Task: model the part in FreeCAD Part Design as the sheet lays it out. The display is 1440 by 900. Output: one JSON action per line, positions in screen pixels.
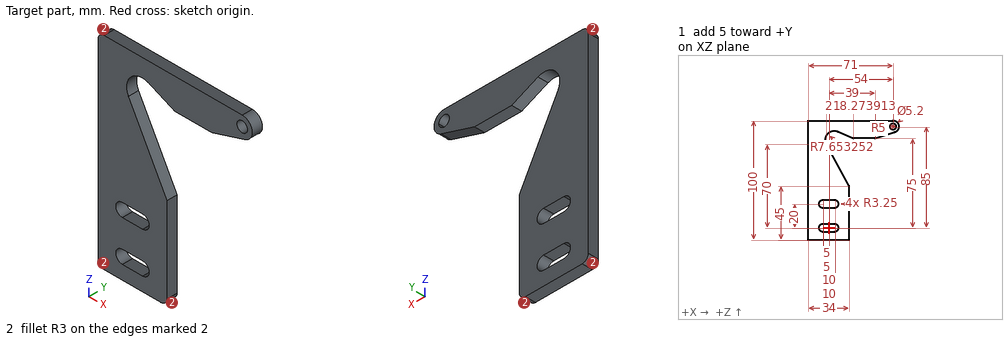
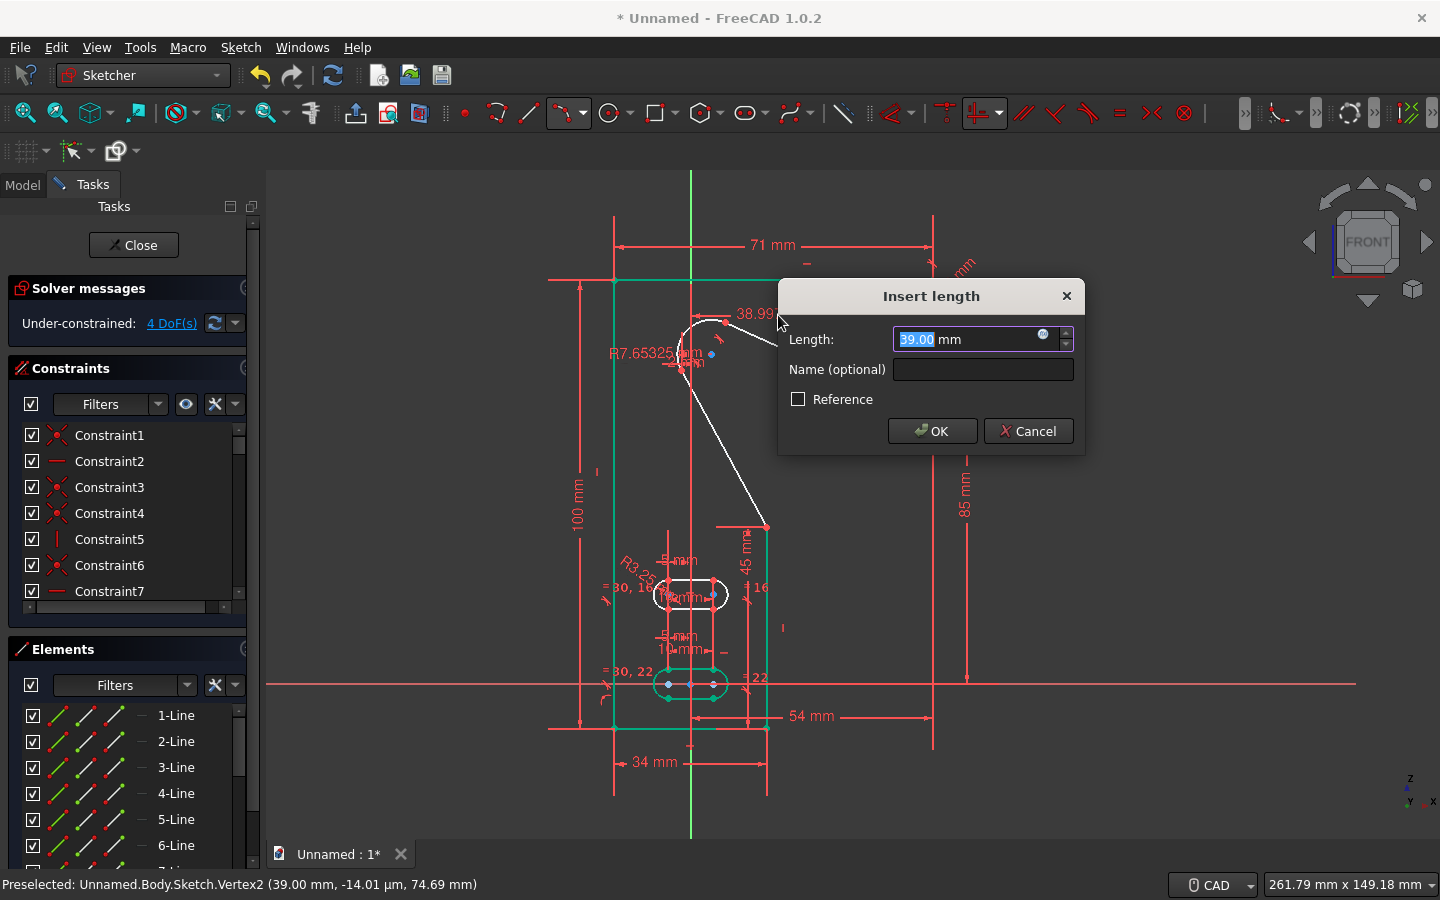
{"action": "type", "text": "39"}
{"action": "key", "text": "Return"}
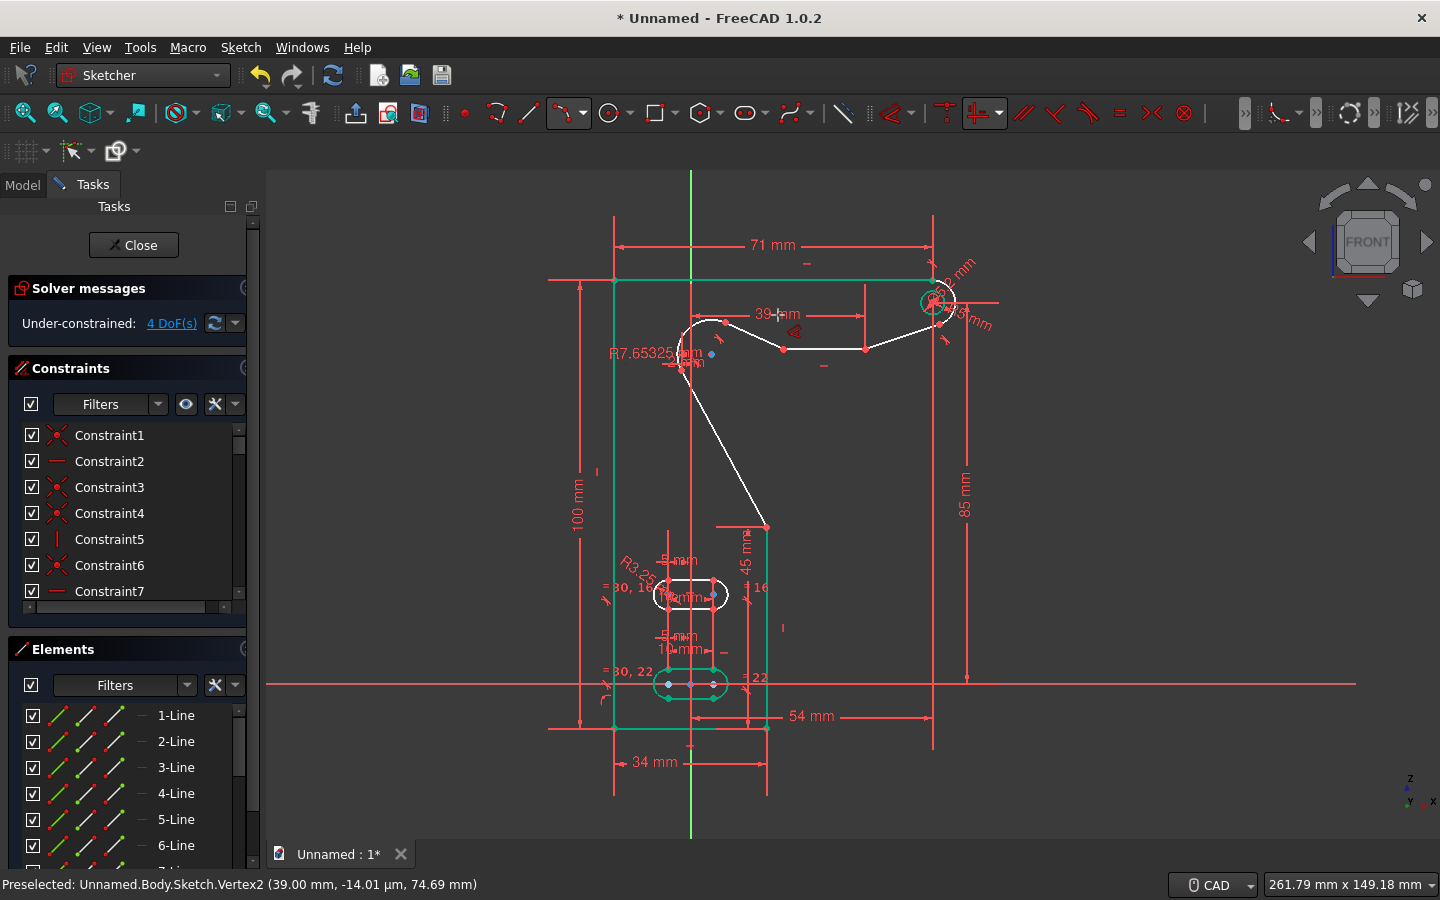
{"action": "left_click", "coordinate": [865, 349]}
{"action": "left_click", "coordinate": [657, 517]}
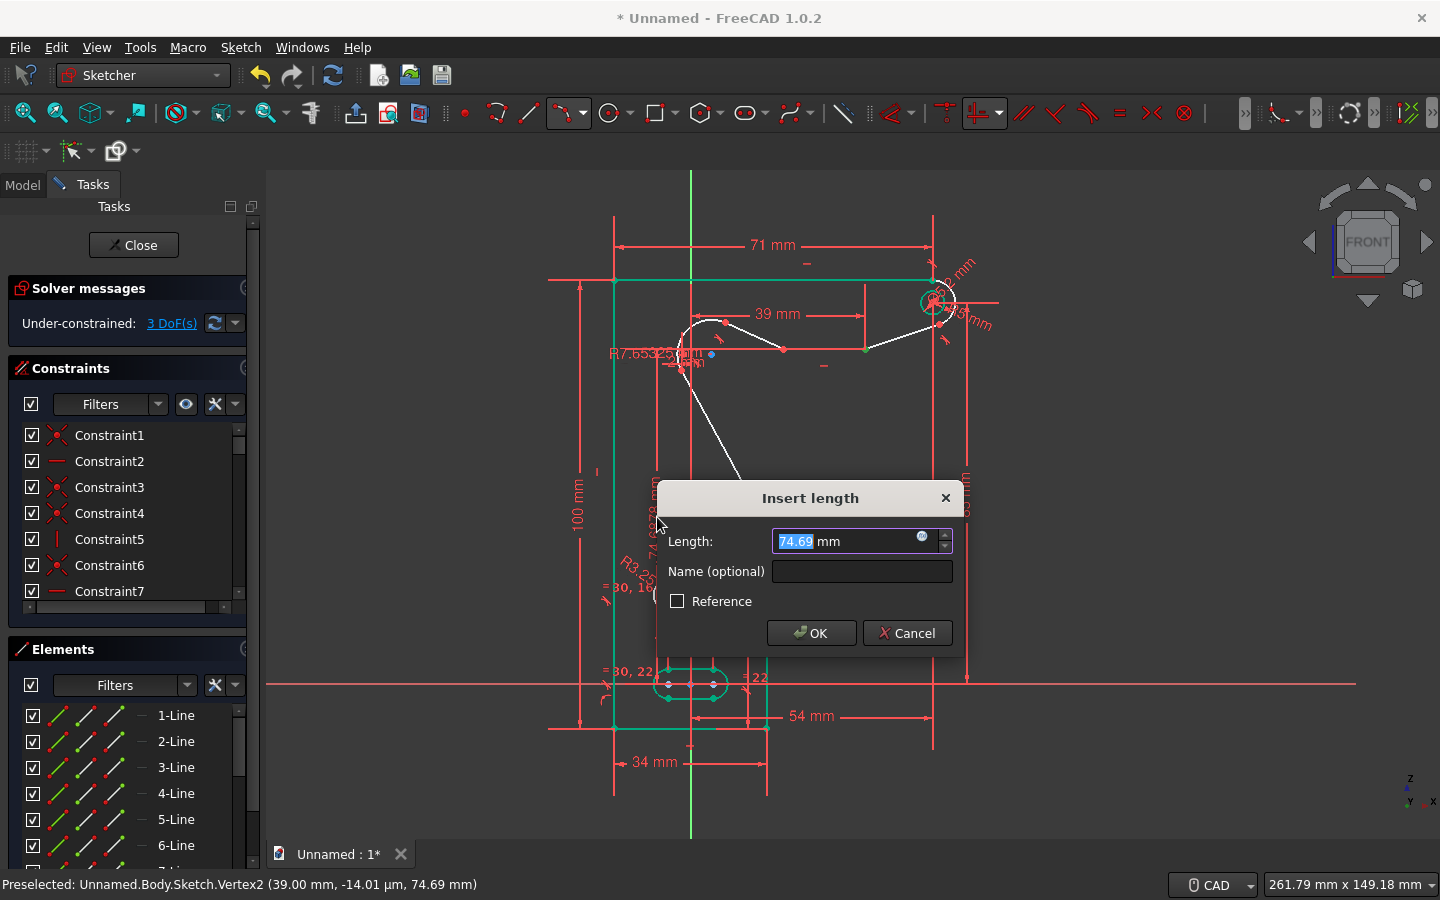
{"action": "type", "text": "75"}
{"action": "key", "text": "Return"}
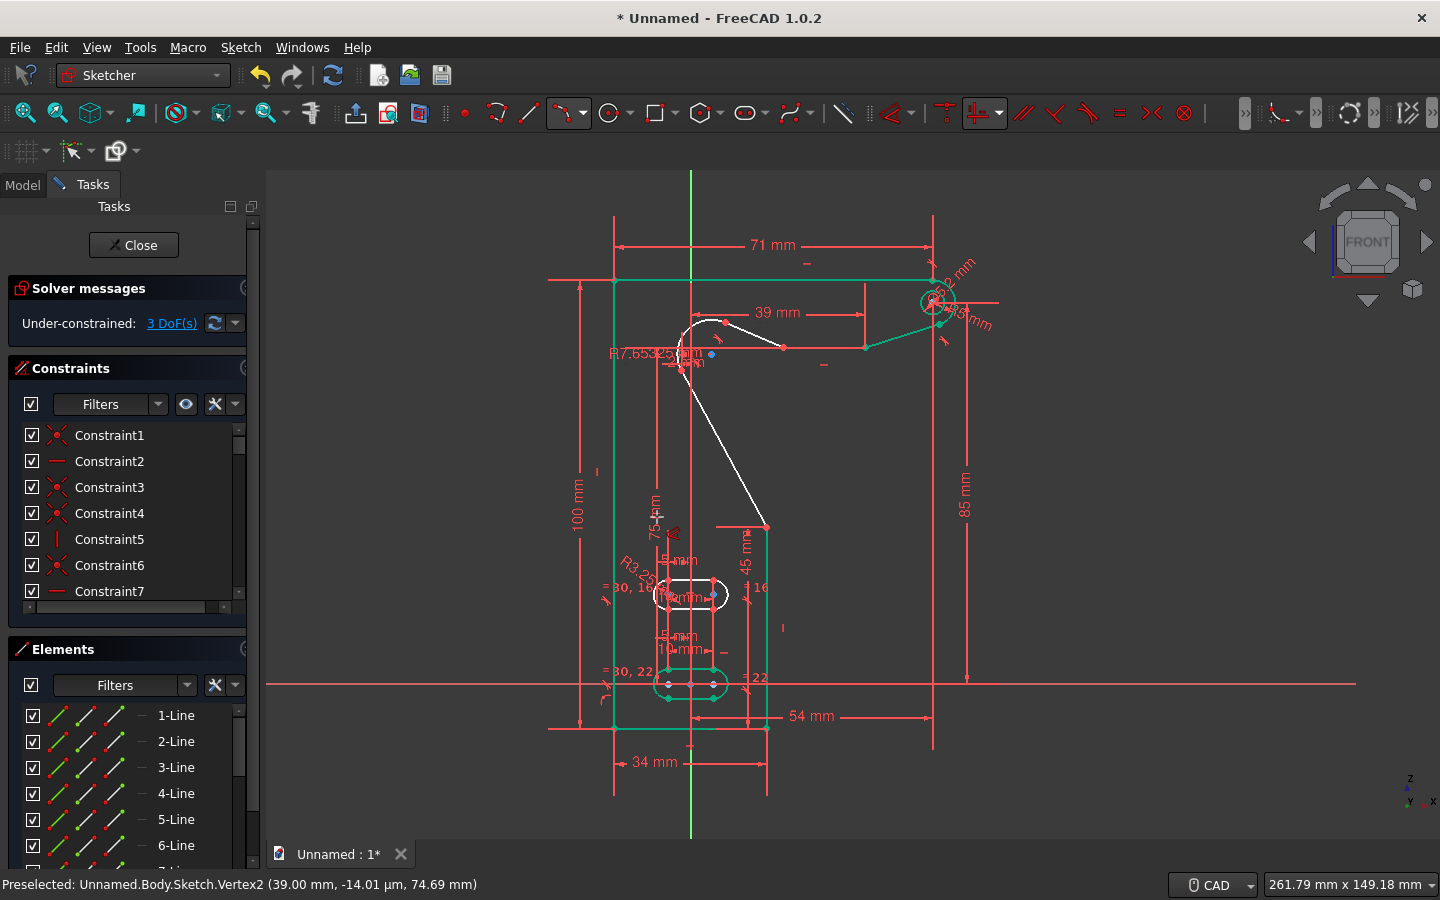
{"action": "left_click", "coordinate": [682, 371]}
{"action": "left_click", "coordinate": [648, 455]}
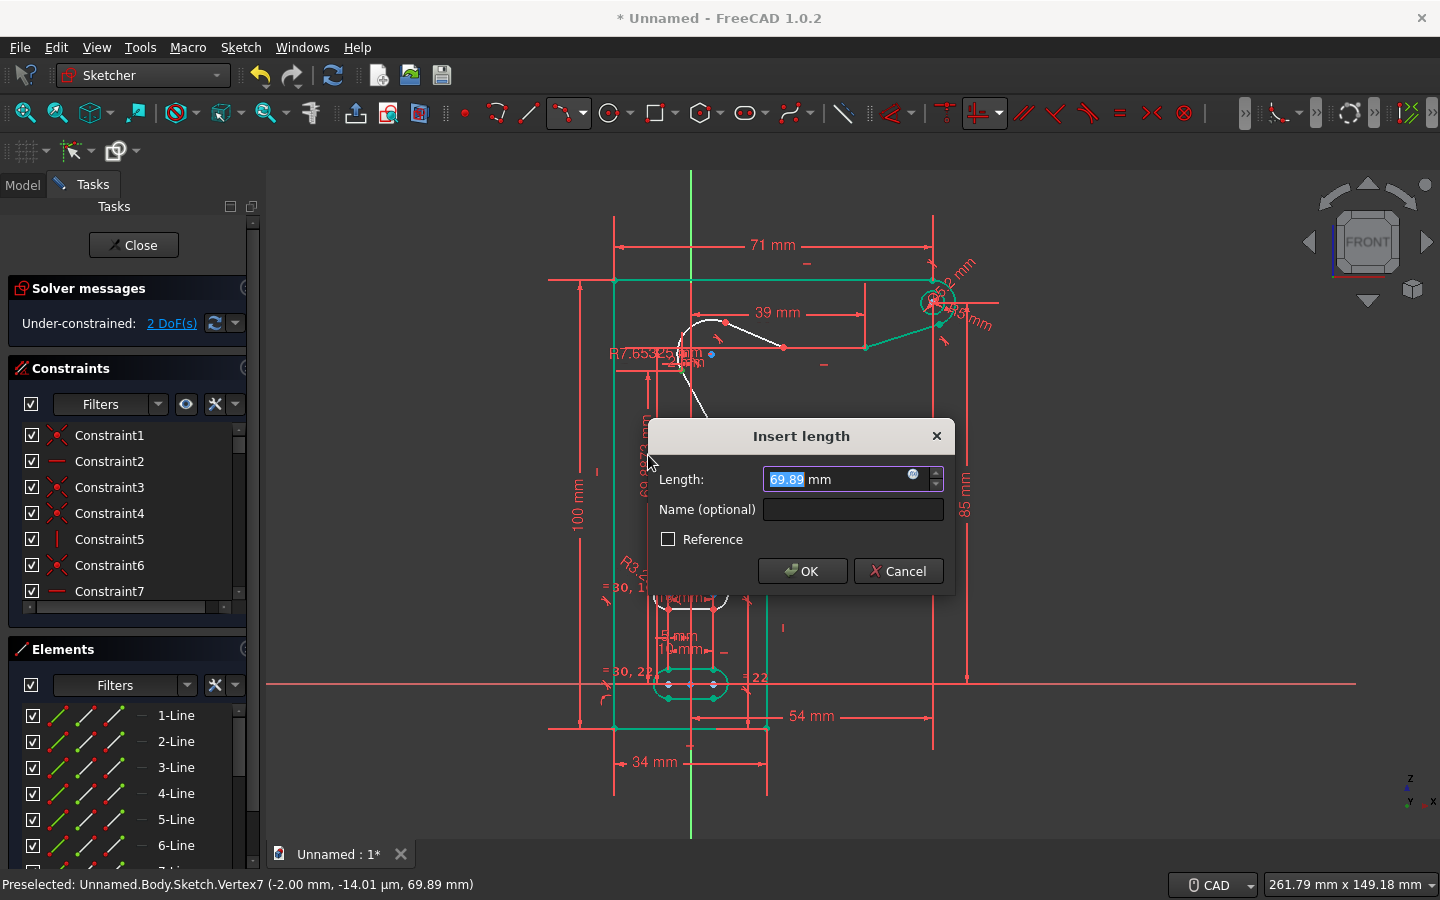
{"action": "type", "text": "70"}
{"action": "key", "text": "Return"}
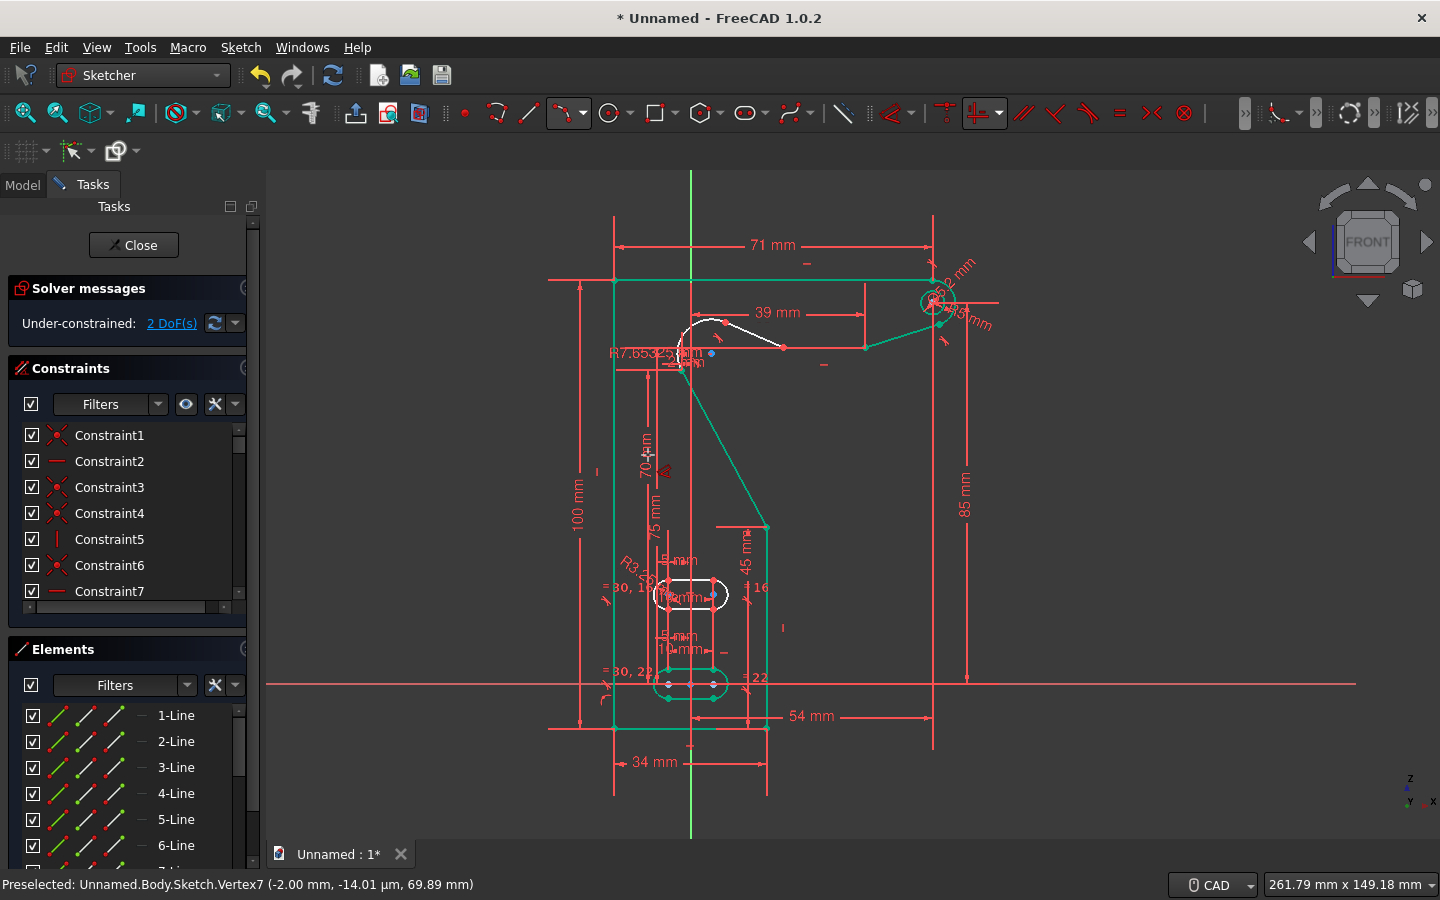
{"action": "left_click", "coordinate": [668, 595]}
{"action": "left_click", "coordinate": [586, 639]}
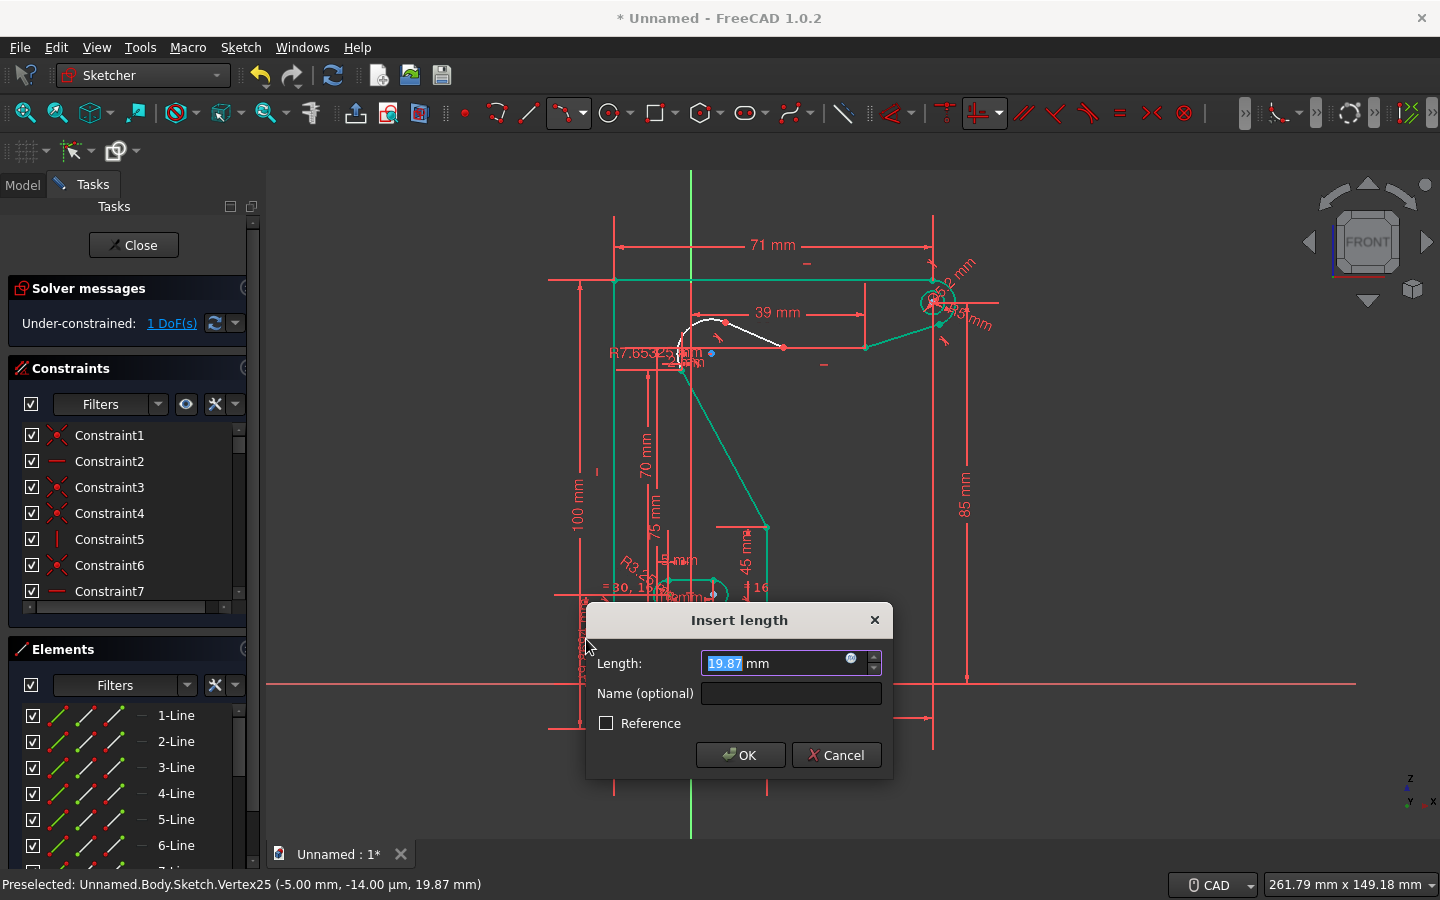
{"action": "type", "text": "20"}
{"action": "key", "text": "Return"}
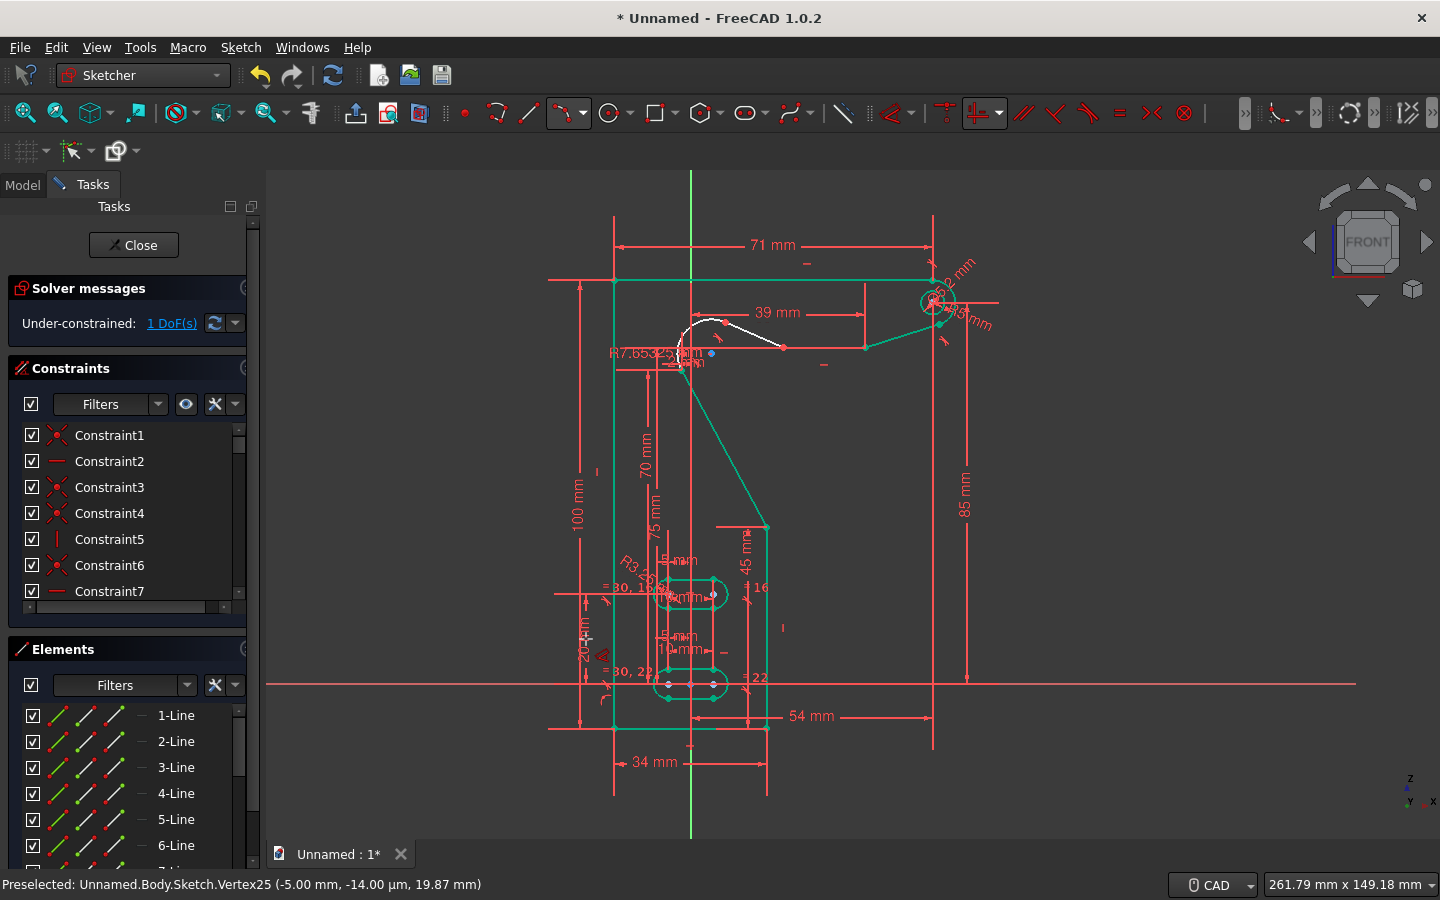
{"action": "left_click", "coordinate": [841, 348]}
{"action": "left_click", "coordinate": [853, 314]}